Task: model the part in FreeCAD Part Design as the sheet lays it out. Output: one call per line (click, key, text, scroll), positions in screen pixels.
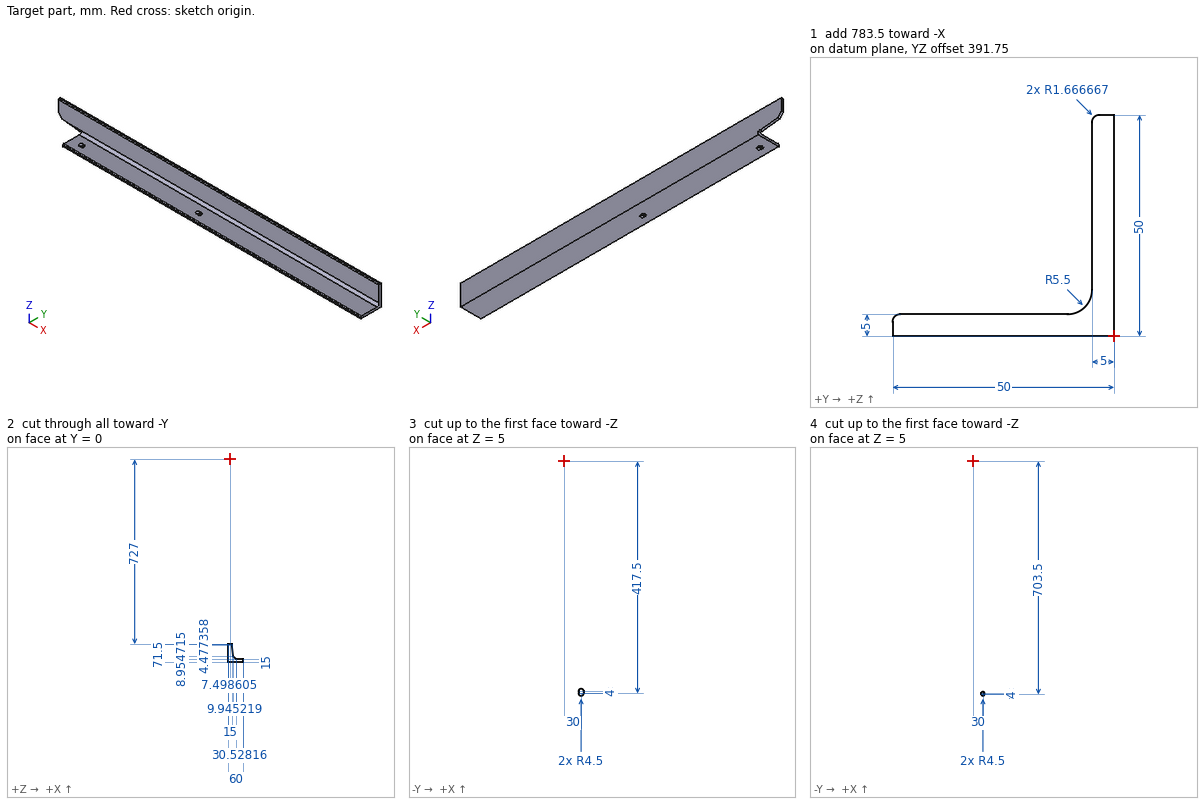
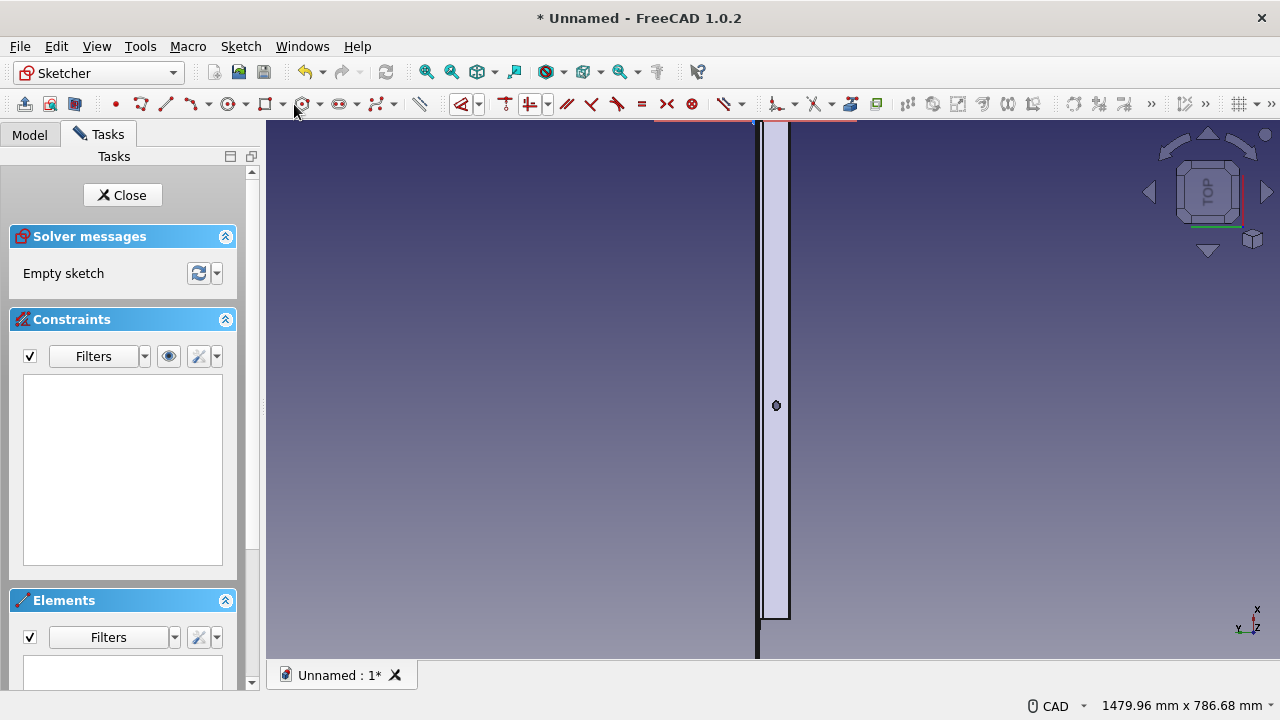
click(75, 104)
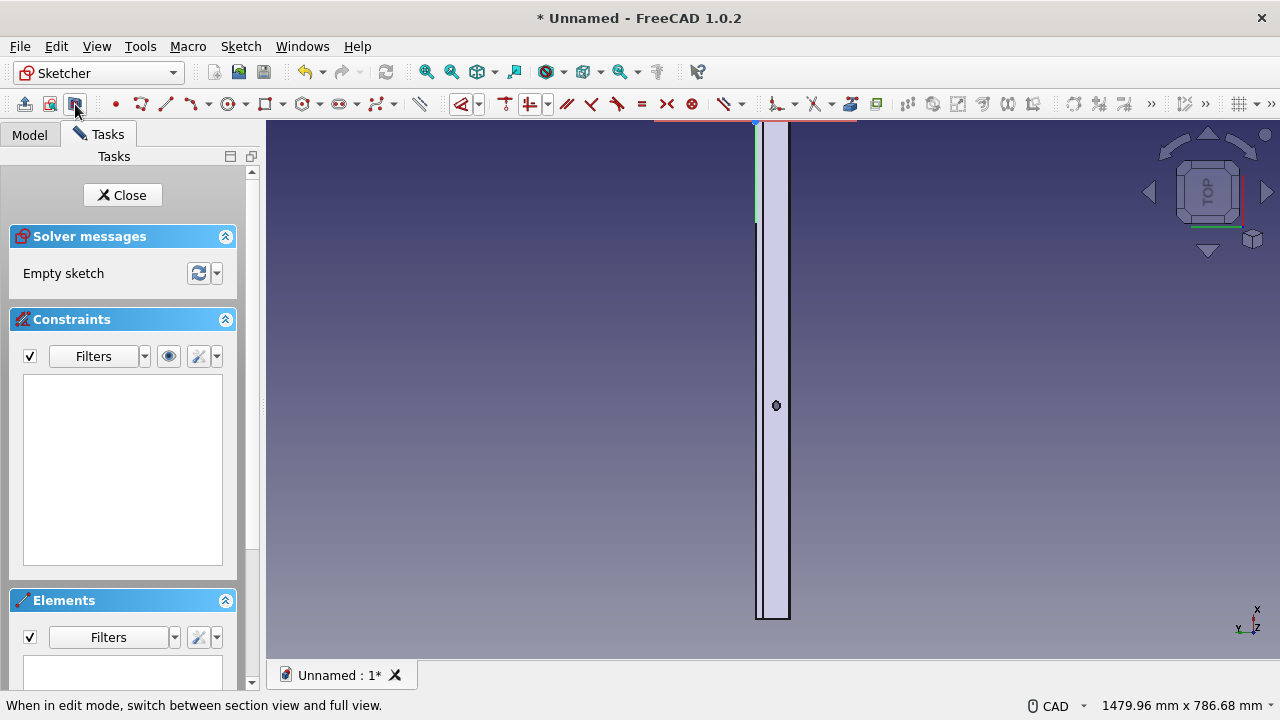
scroll(780, 613, up, 15)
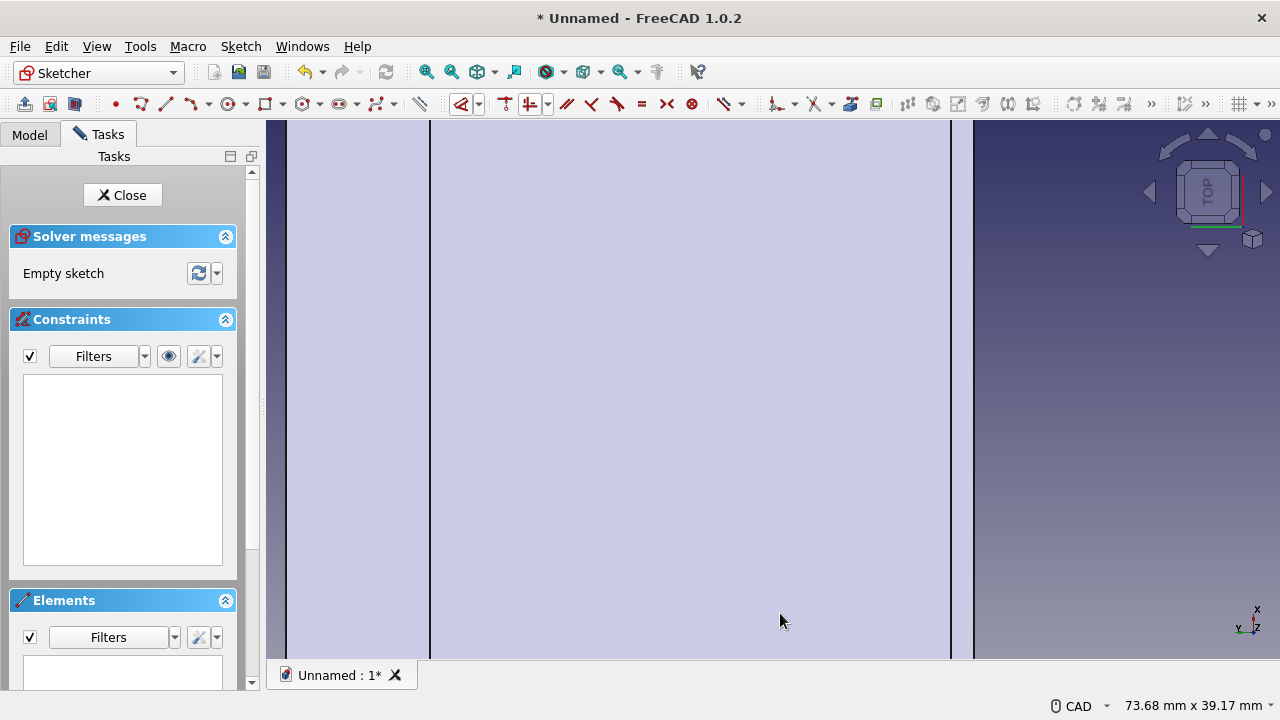
scroll(691, 344, up, 3)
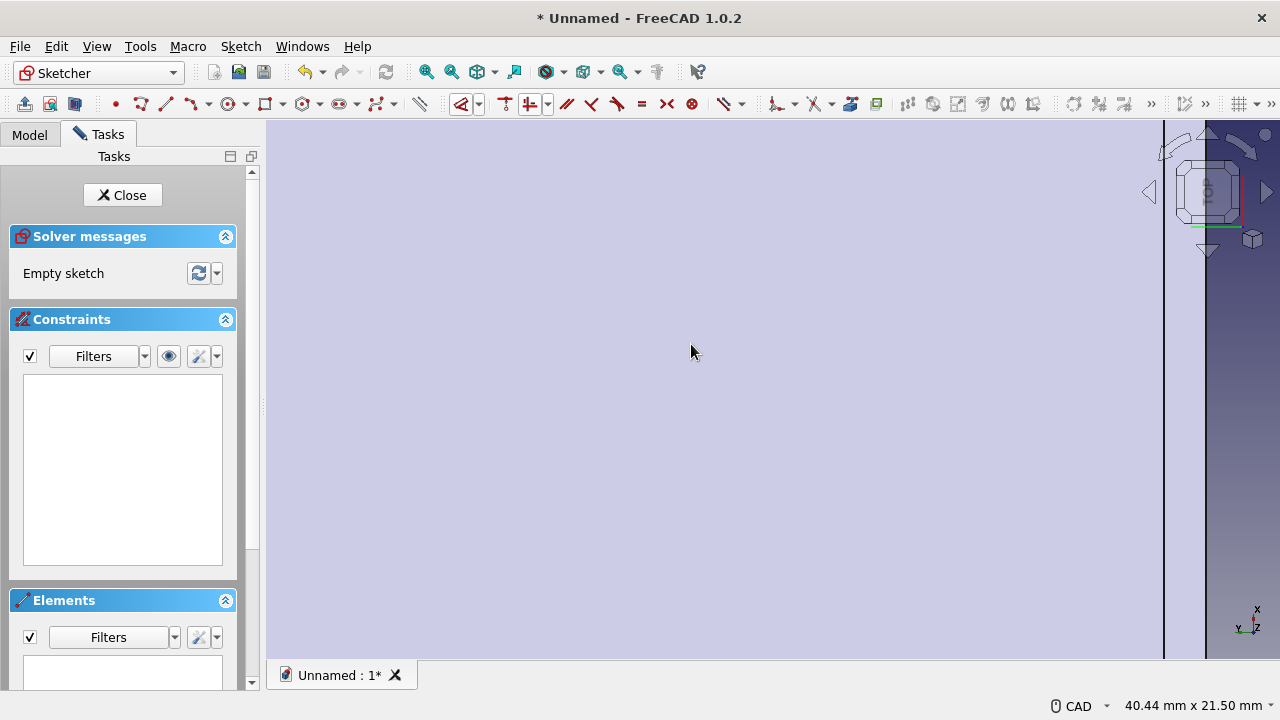
click(338, 104)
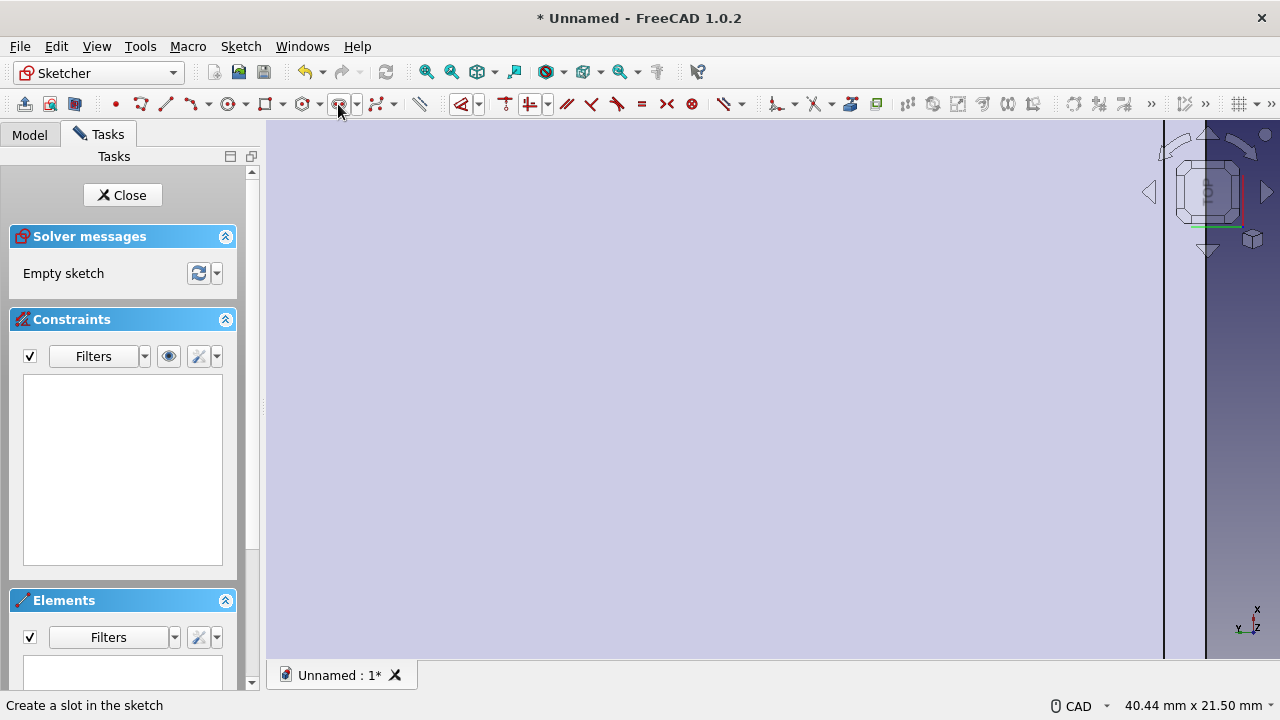
click(704, 440)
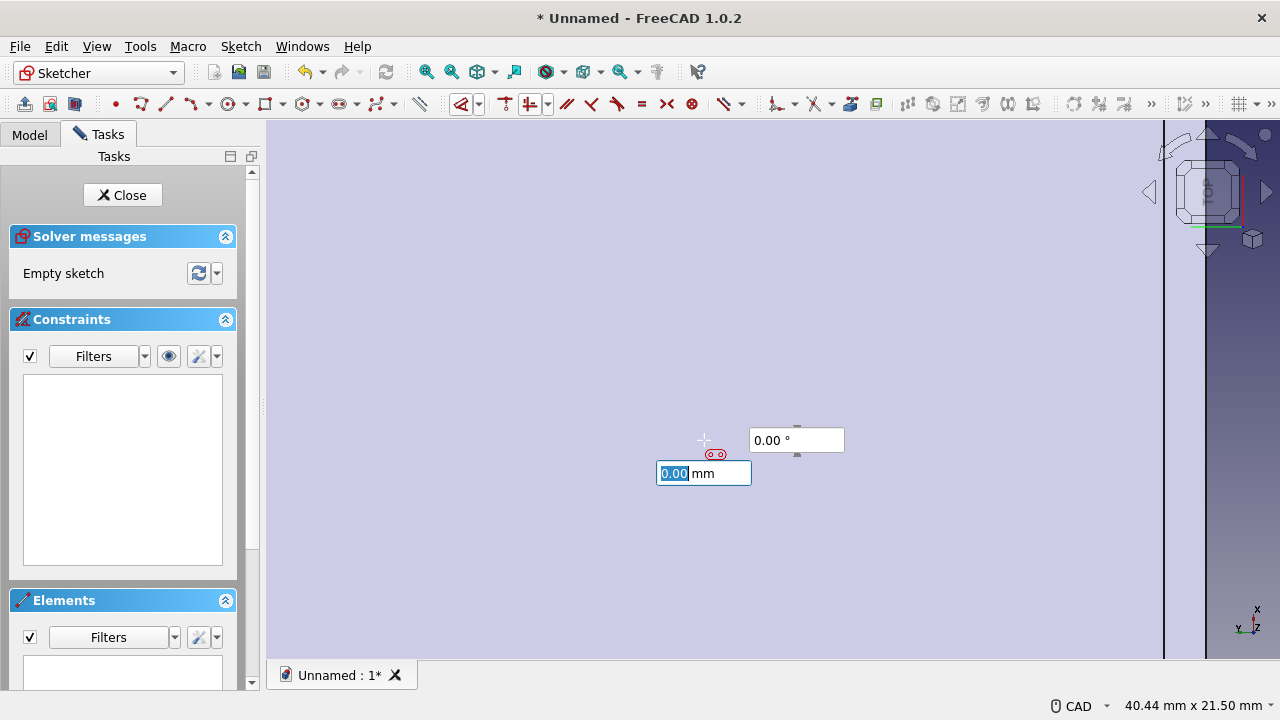
click(704, 339)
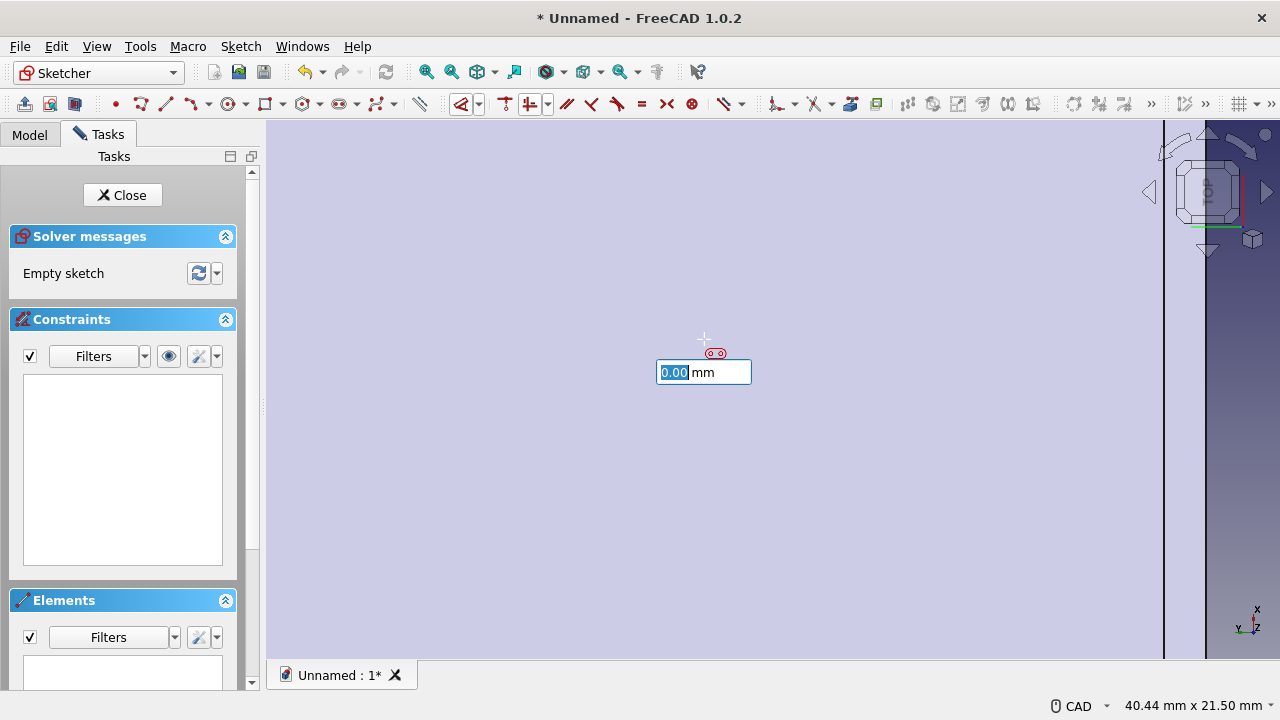
click(592, 389)
key(Escape)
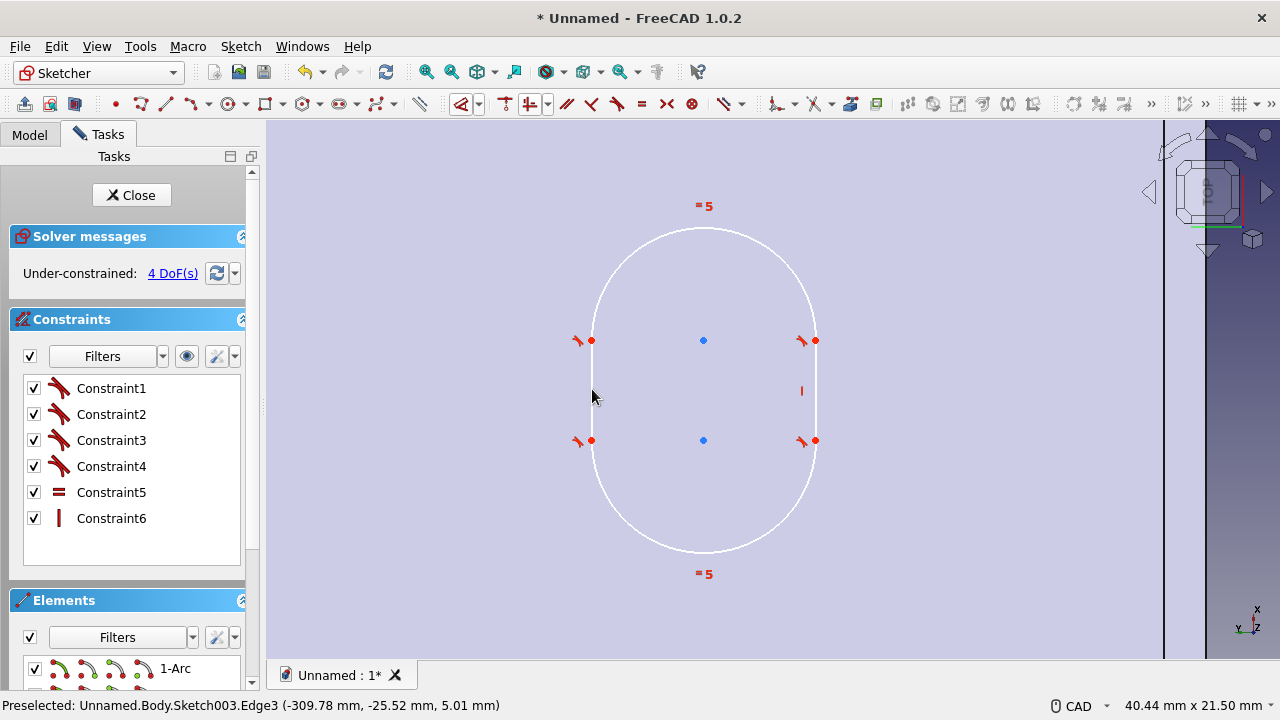
click(638, 532)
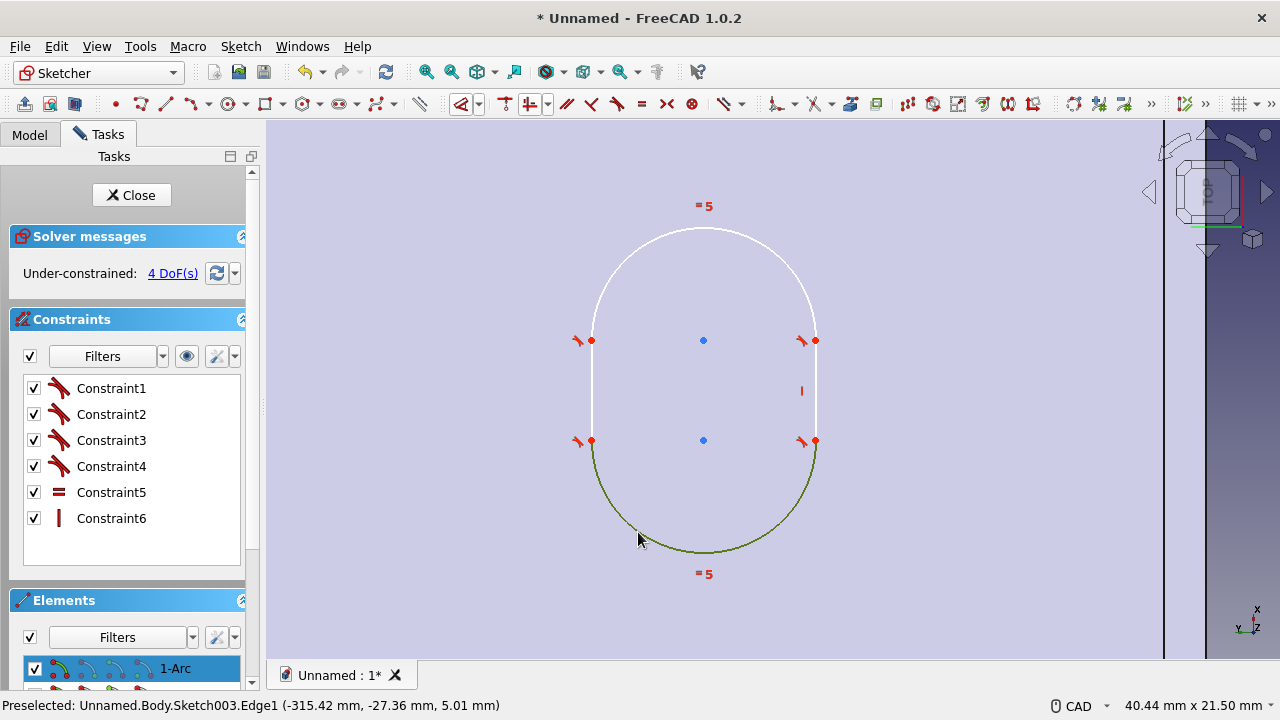
key(k)
key(r)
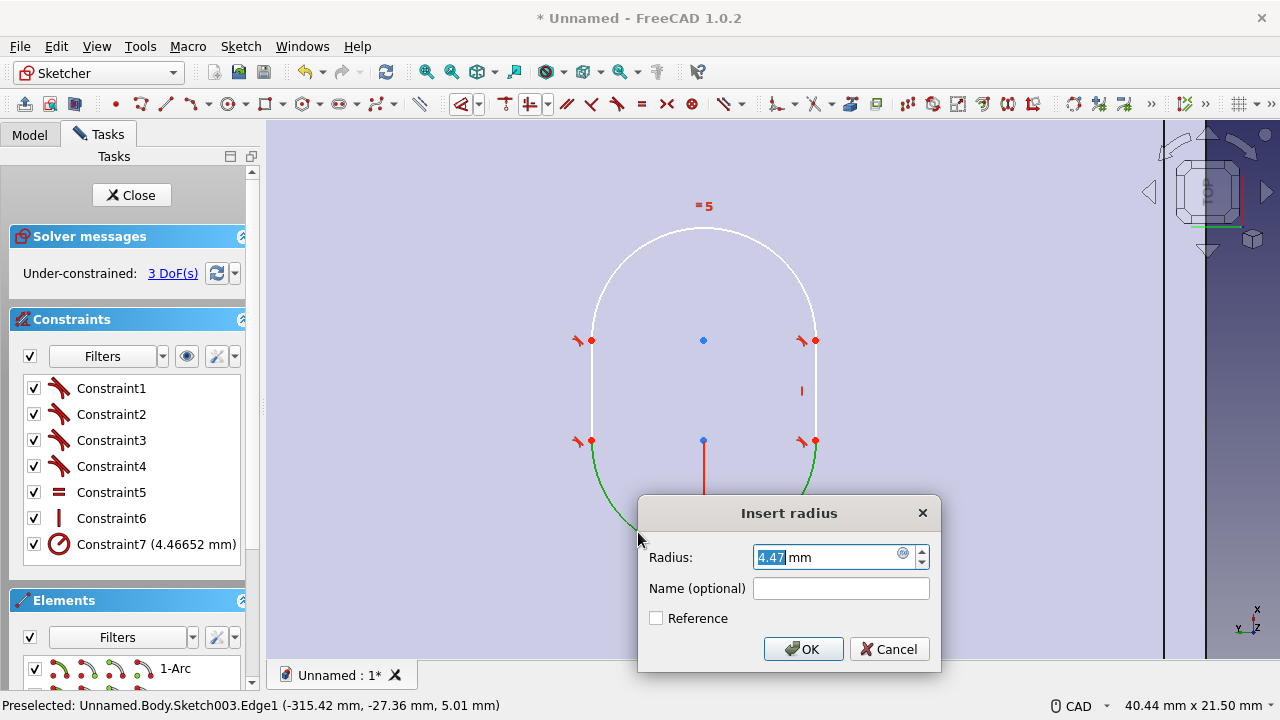
text(4.5)
key(Return)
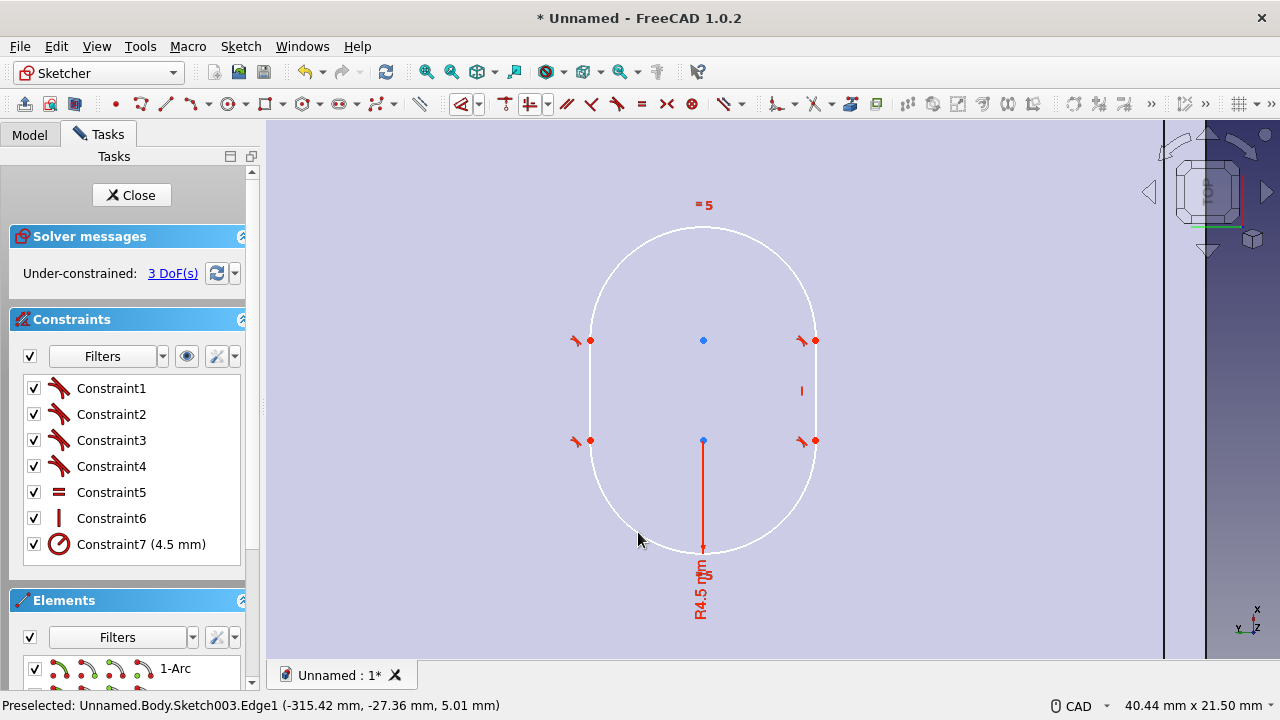
click(590, 411)